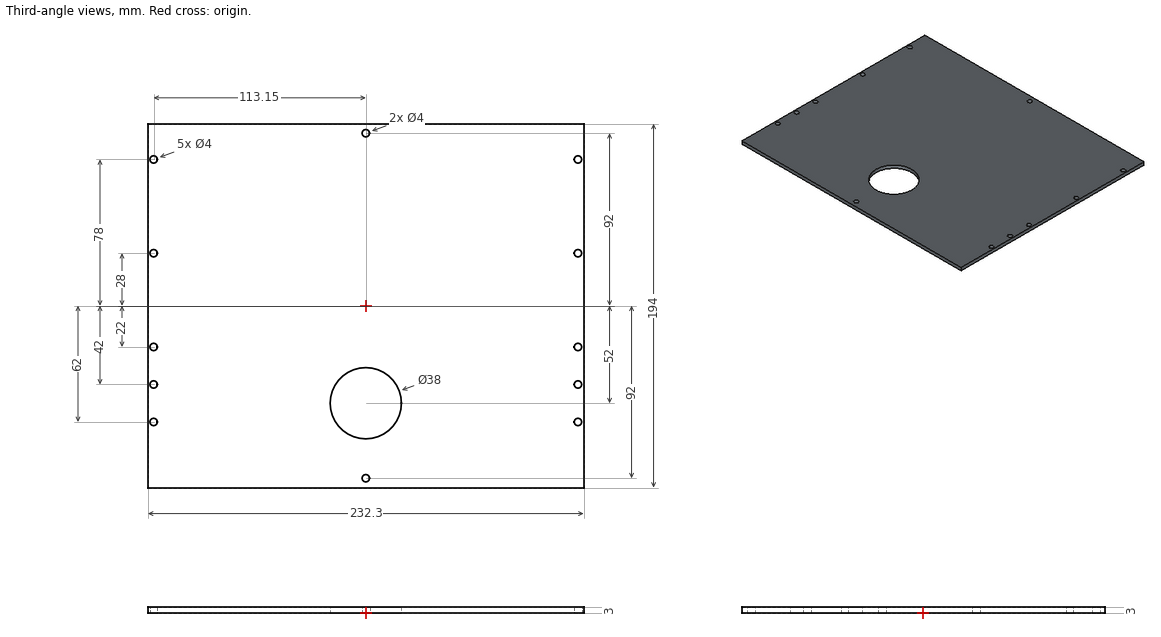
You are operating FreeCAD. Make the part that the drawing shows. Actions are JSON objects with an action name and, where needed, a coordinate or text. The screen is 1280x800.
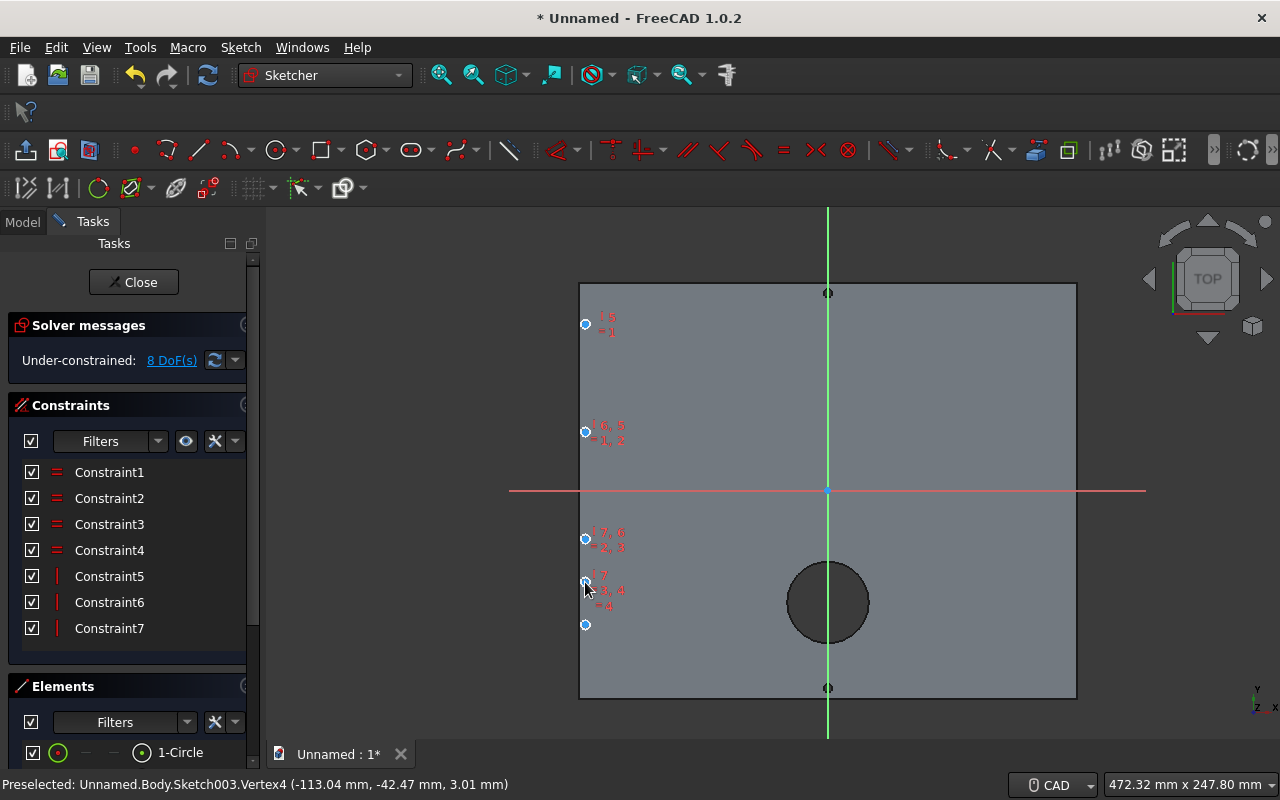
{"action": "left_click", "coordinate": [585, 582]}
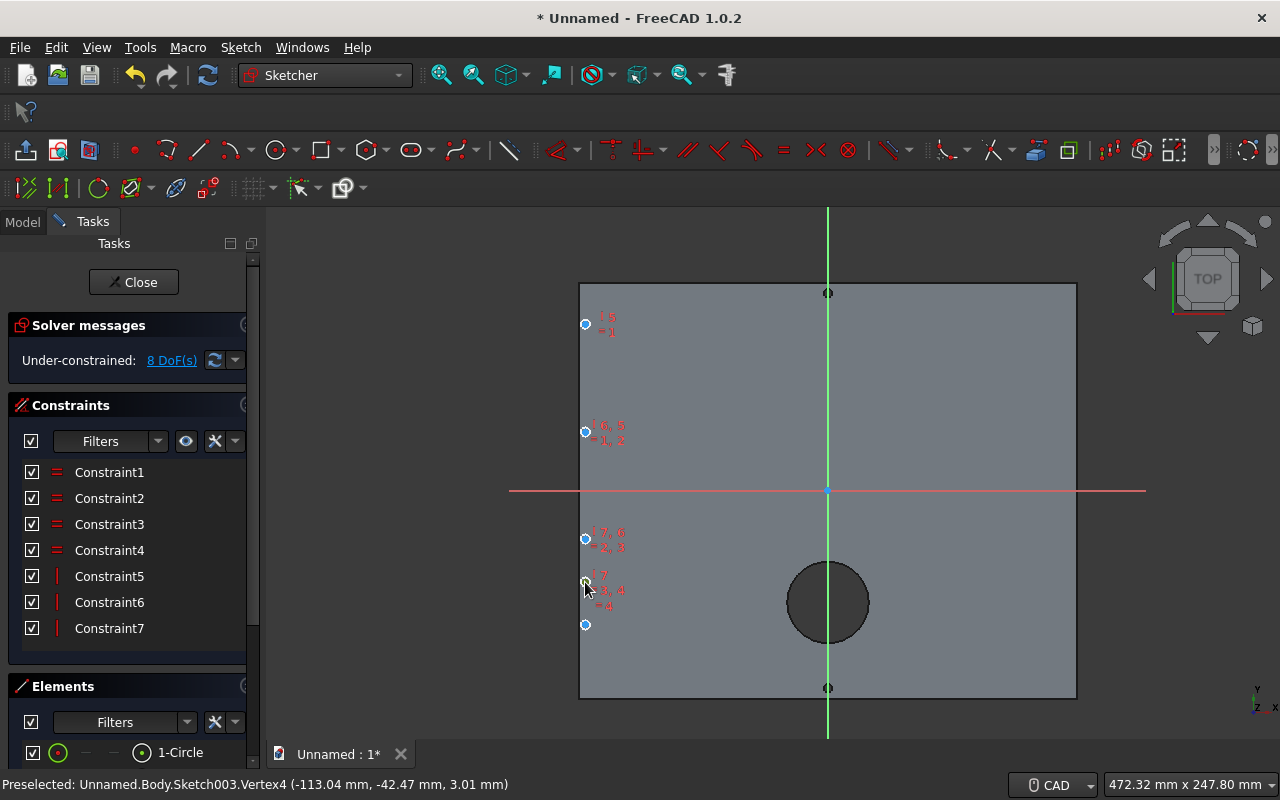
{"action": "left_click", "coordinate": [585, 625]}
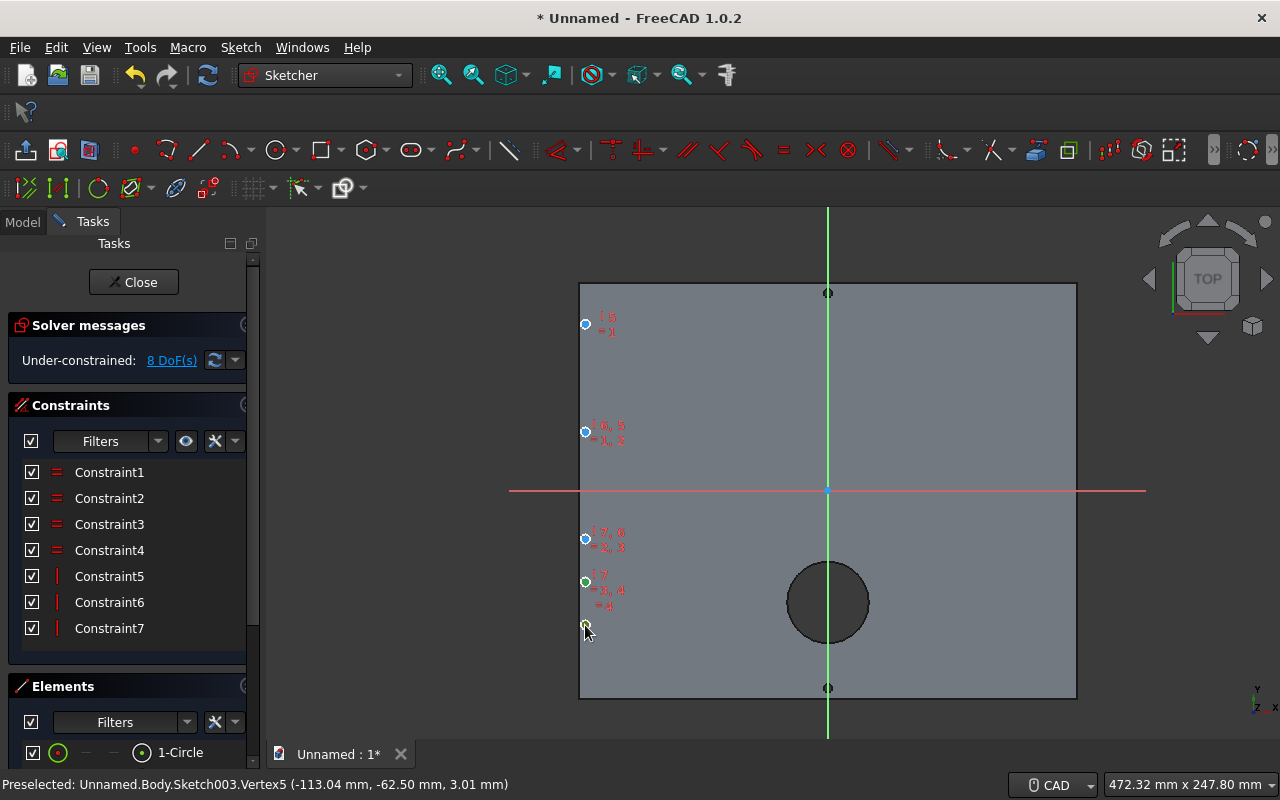
{"action": "key", "text": "v"}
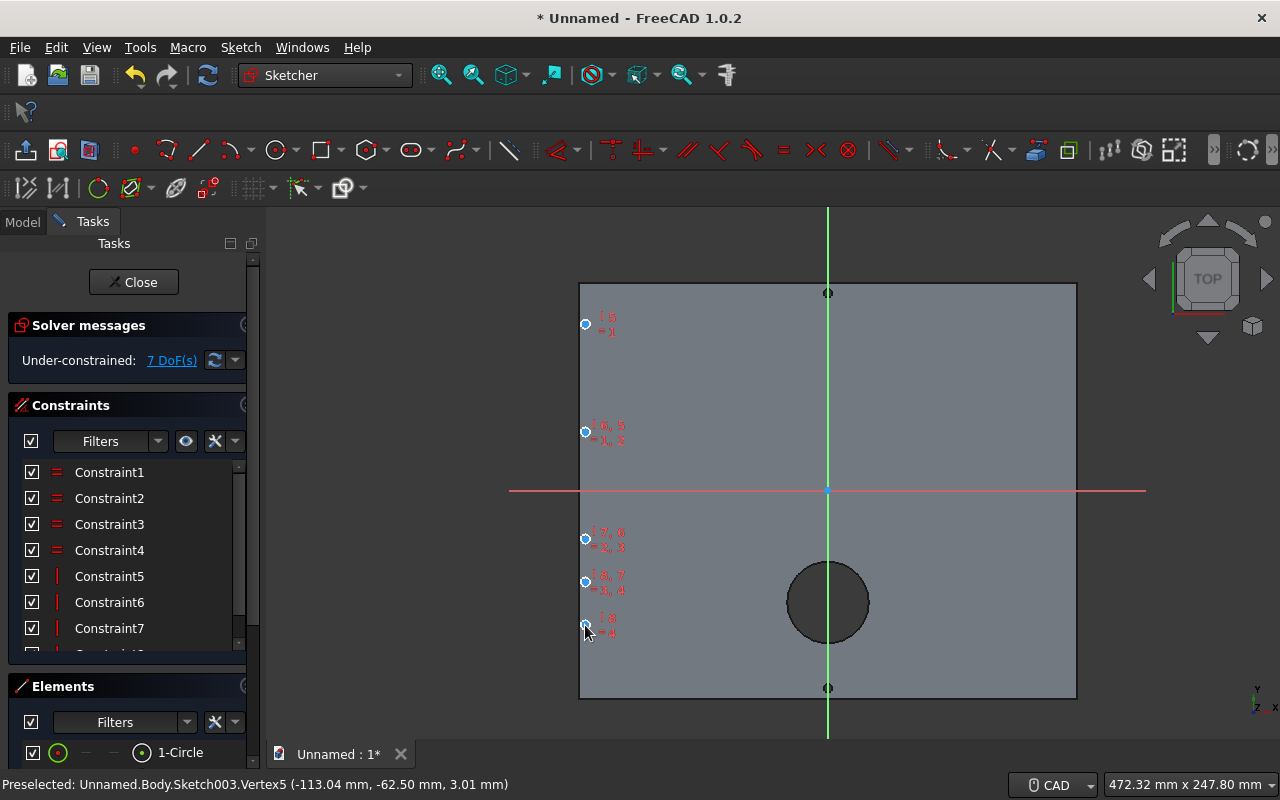
{"action": "key", "text": "d"}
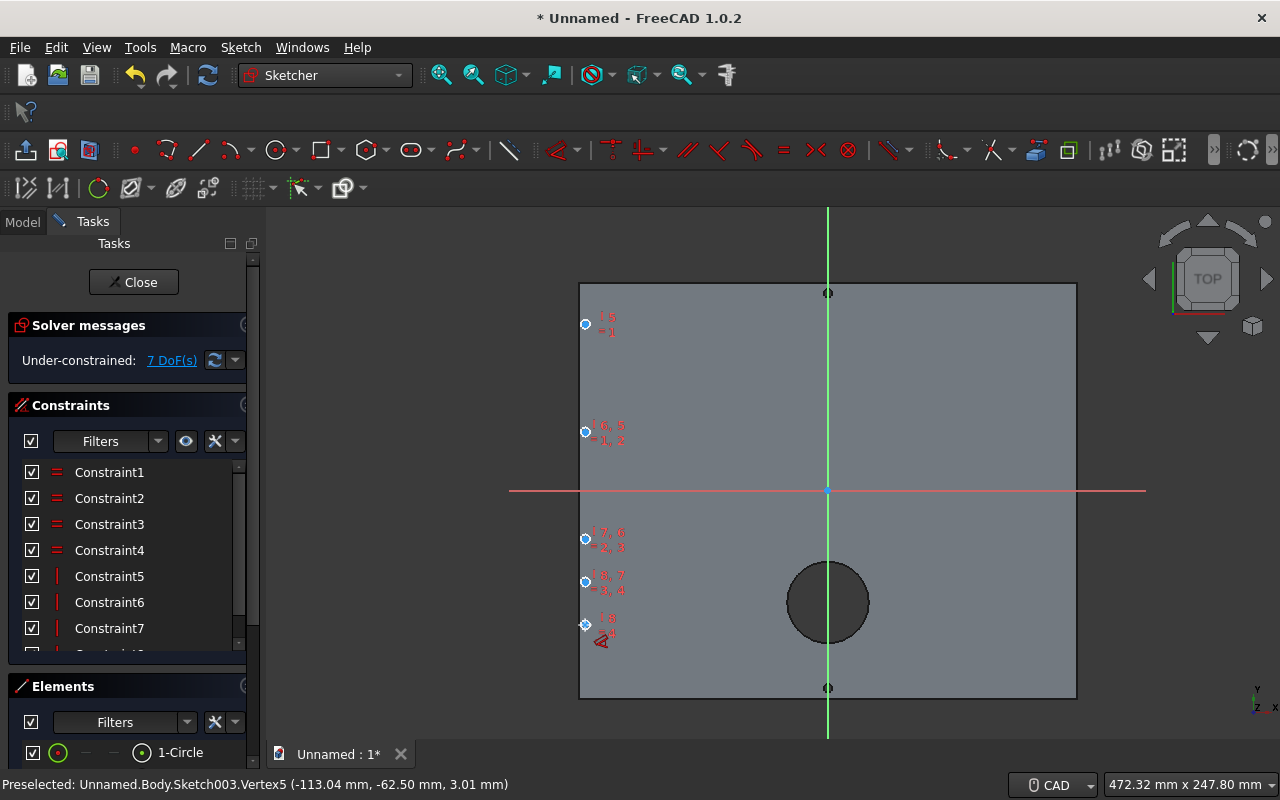
{"action": "scroll", "coordinate": [585, 320], "scroll_direction": "up", "scroll_amount": 8}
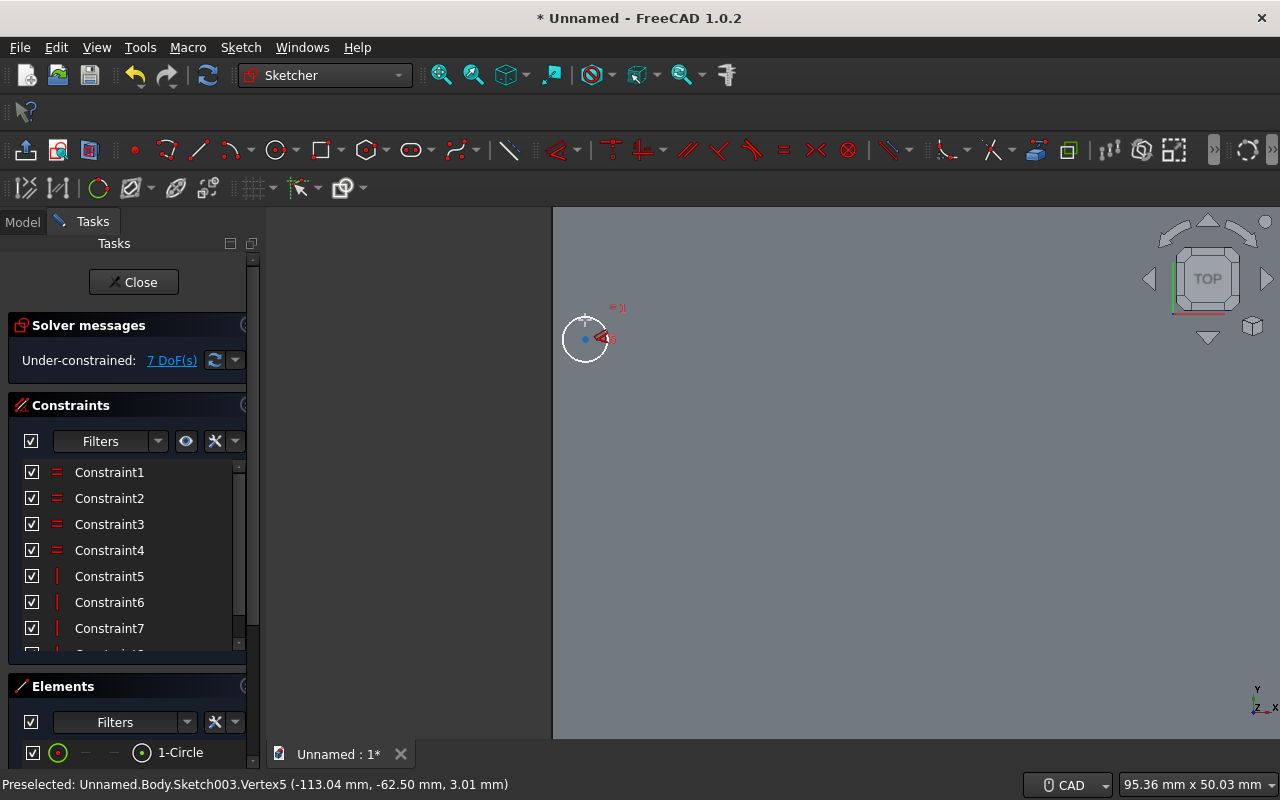
{"action": "left_click", "coordinate": [586, 317]}
{"action": "left_click", "coordinate": [587, 285]}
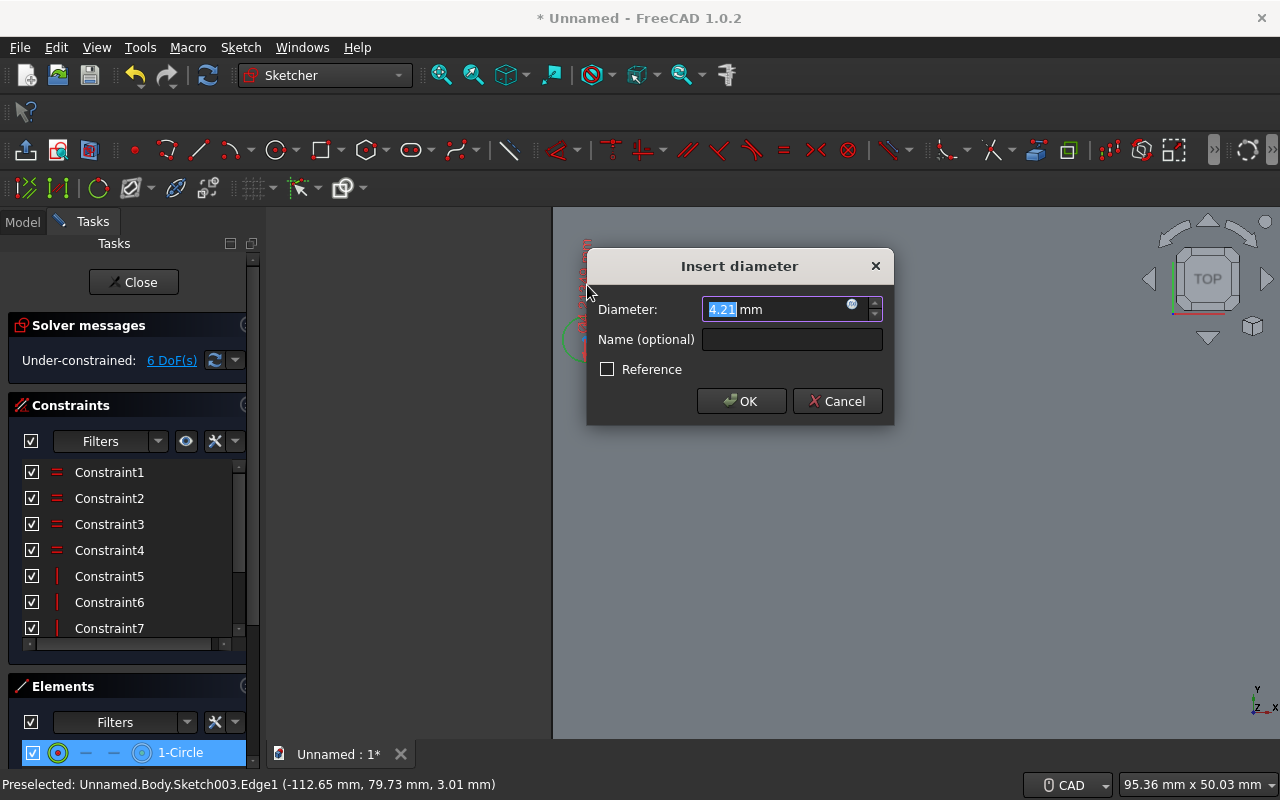
{"action": "type", "text": "4"}
{"action": "key", "text": "Return"}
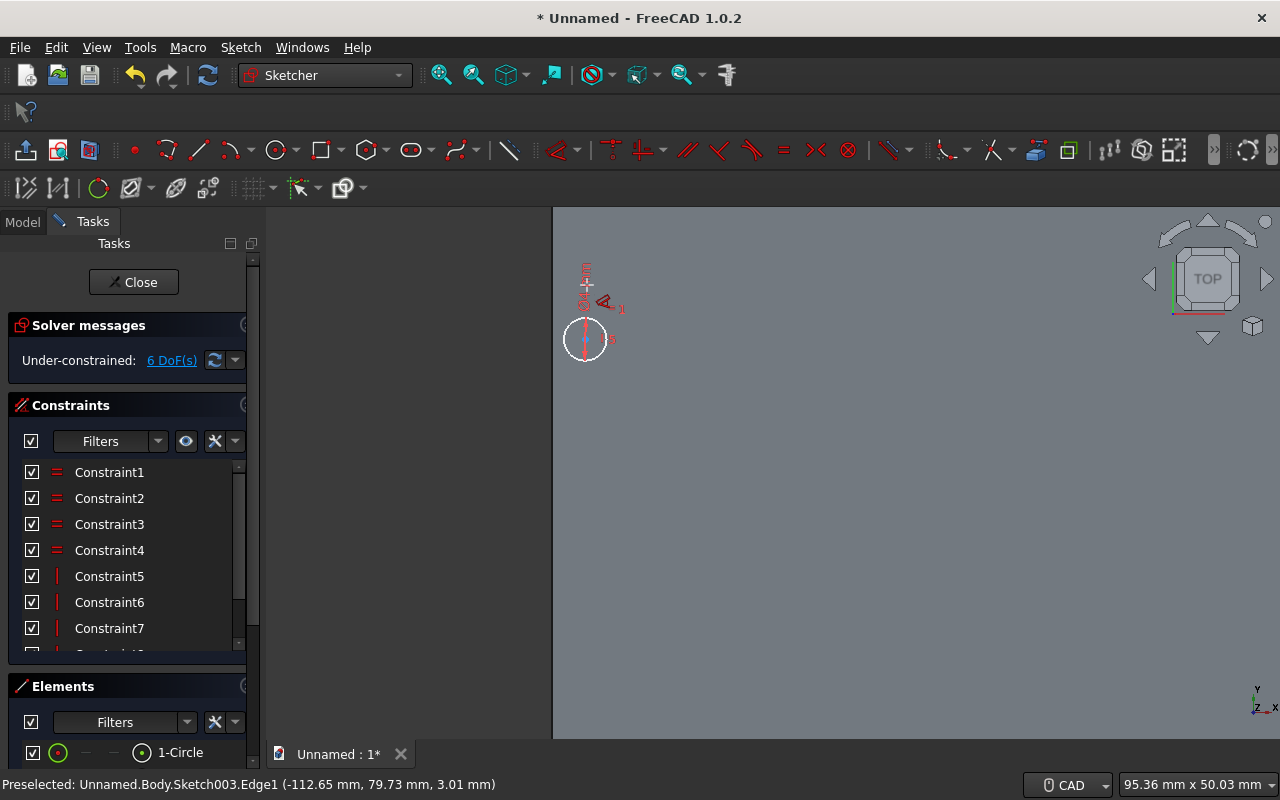
{"action": "scroll", "coordinate": [585, 319], "scroll_direction": "down", "scroll_amount": 8}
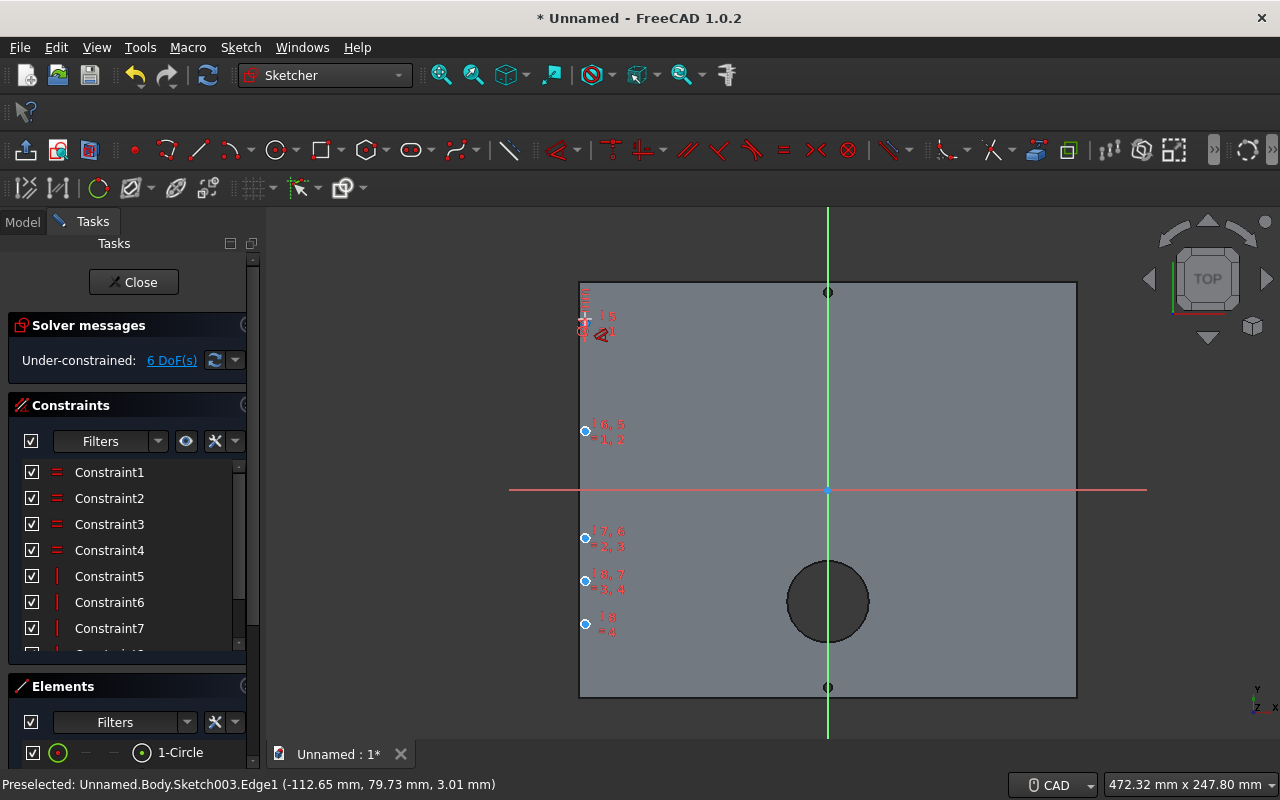
{"action": "left_click", "coordinate": [585, 323]}
{"action": "left_click", "coordinate": [862, 407]}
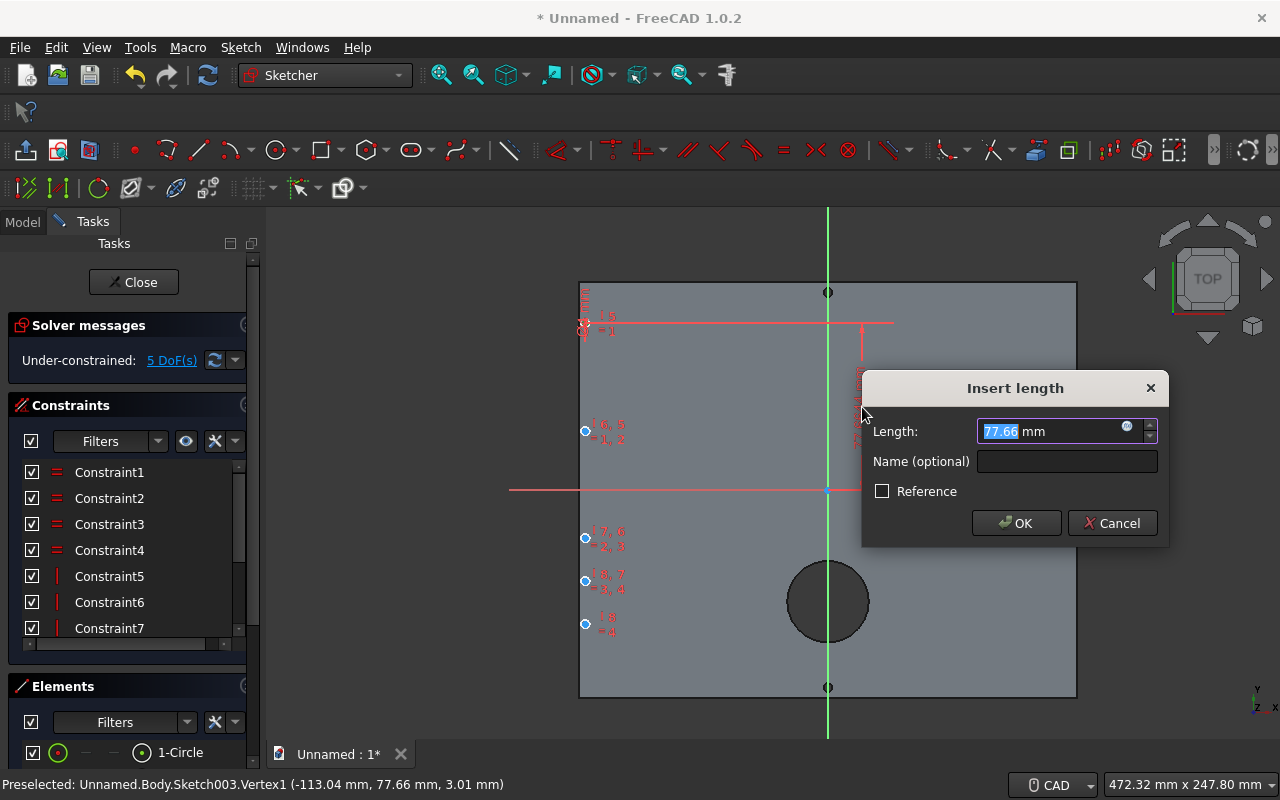
{"action": "type", "text": "78"}
{"action": "key", "text": "Return"}